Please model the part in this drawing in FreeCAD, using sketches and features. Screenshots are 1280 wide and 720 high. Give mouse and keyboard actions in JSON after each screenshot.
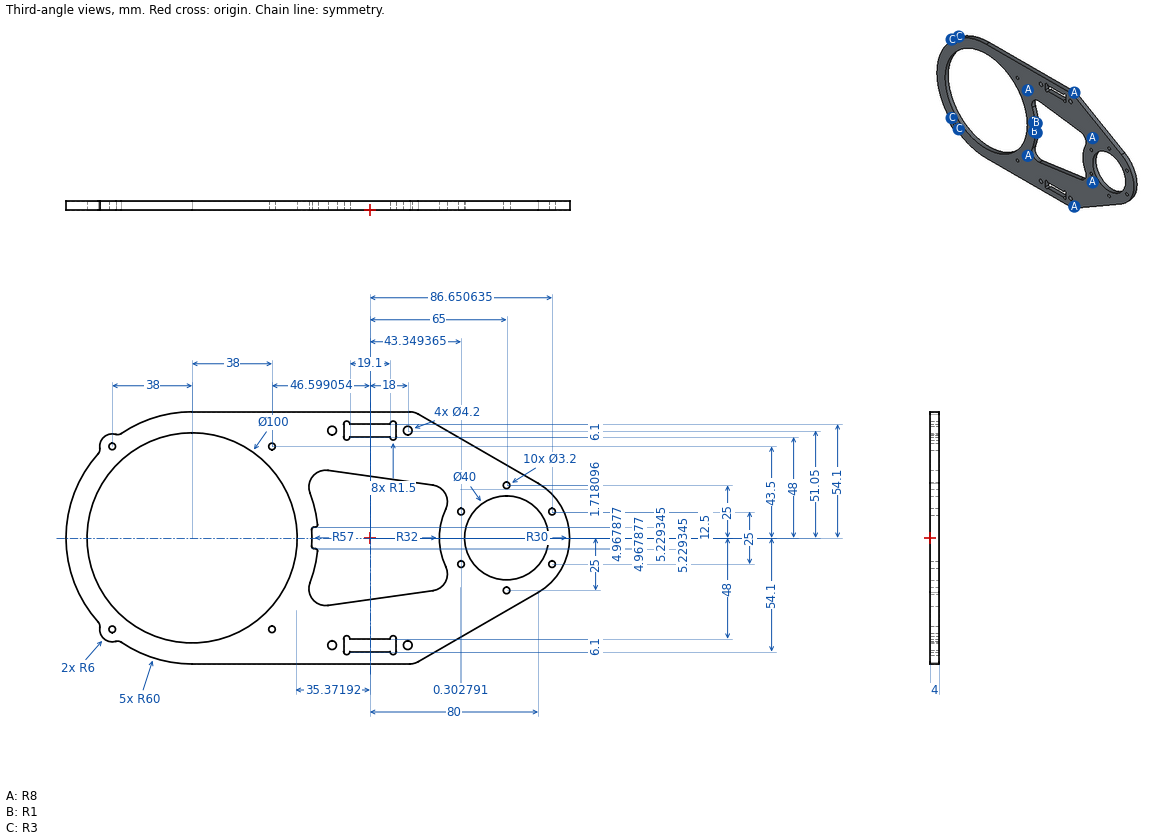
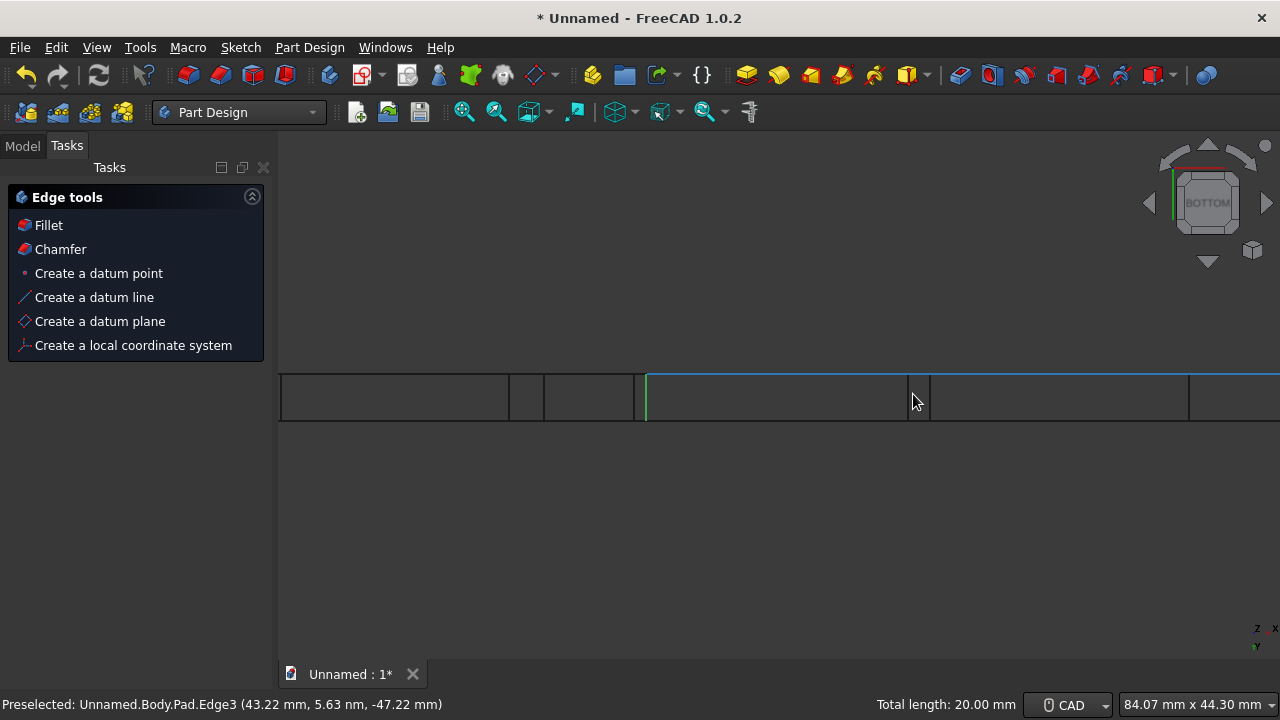
{"action": "left_click", "coordinate": [908, 397], "text": "ctrl"}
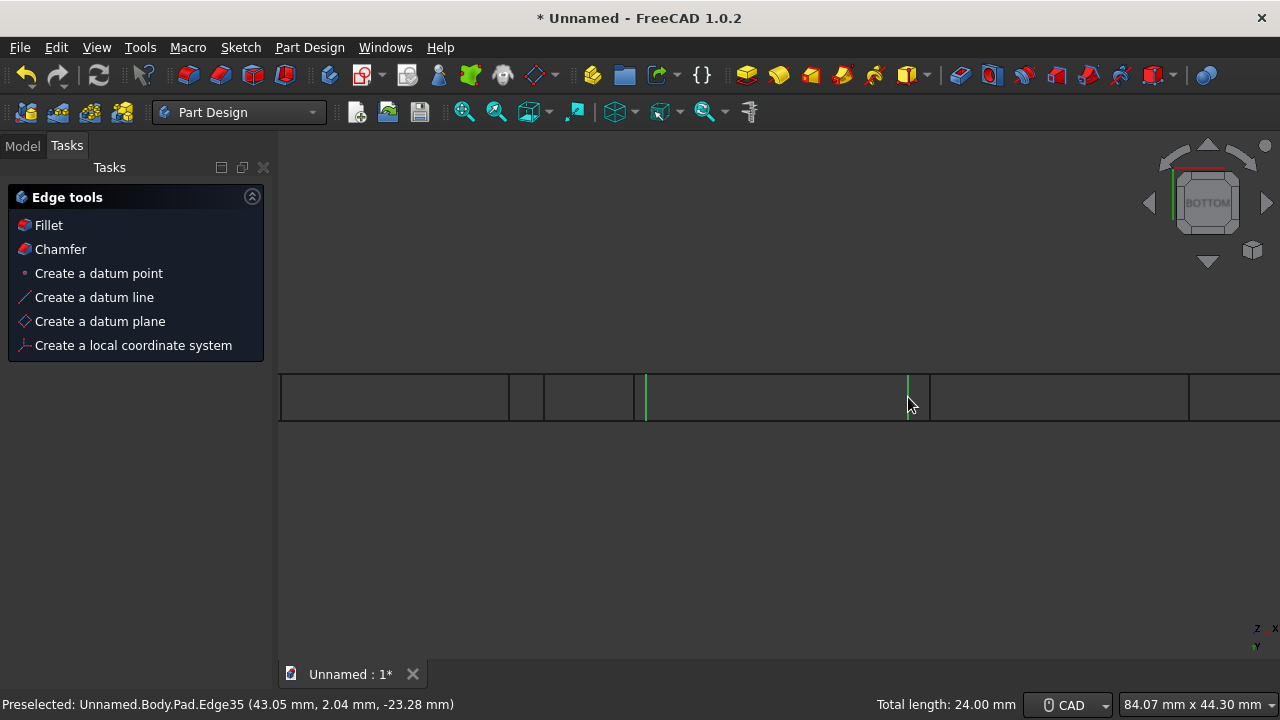
{"action": "key", "text": "v 1"}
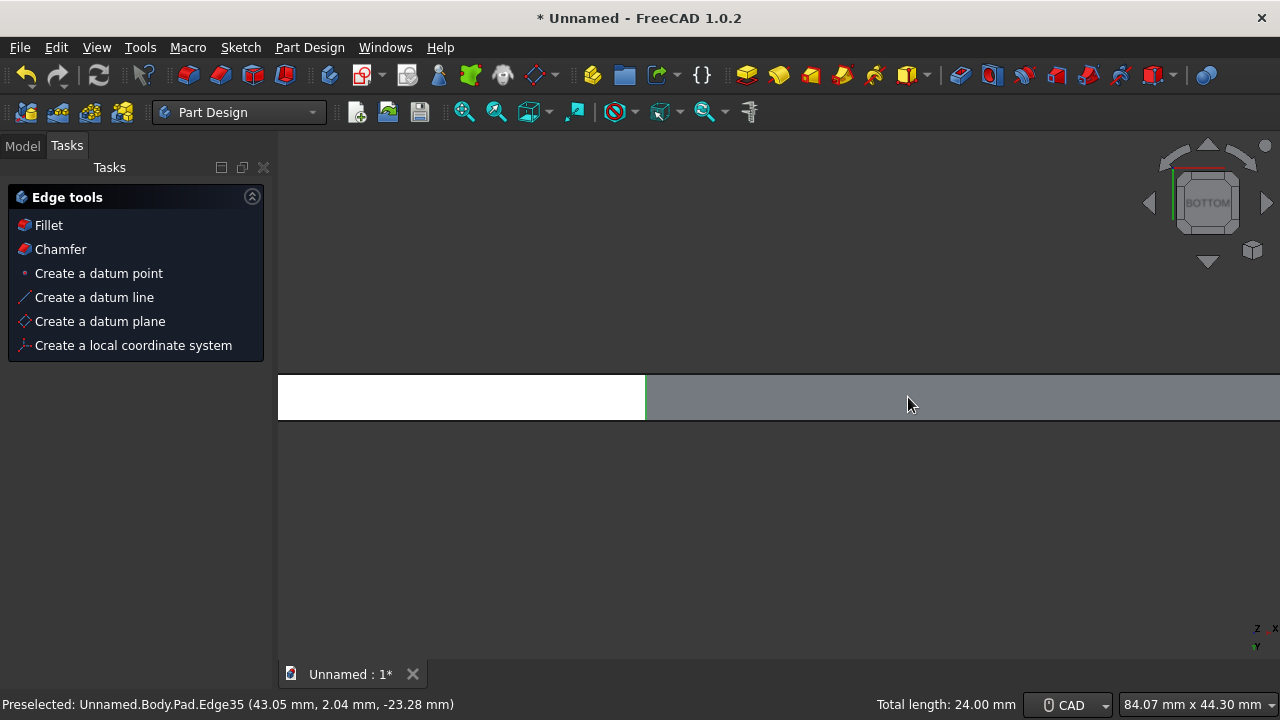
{"action": "left_click", "coordinate": [190, 76]}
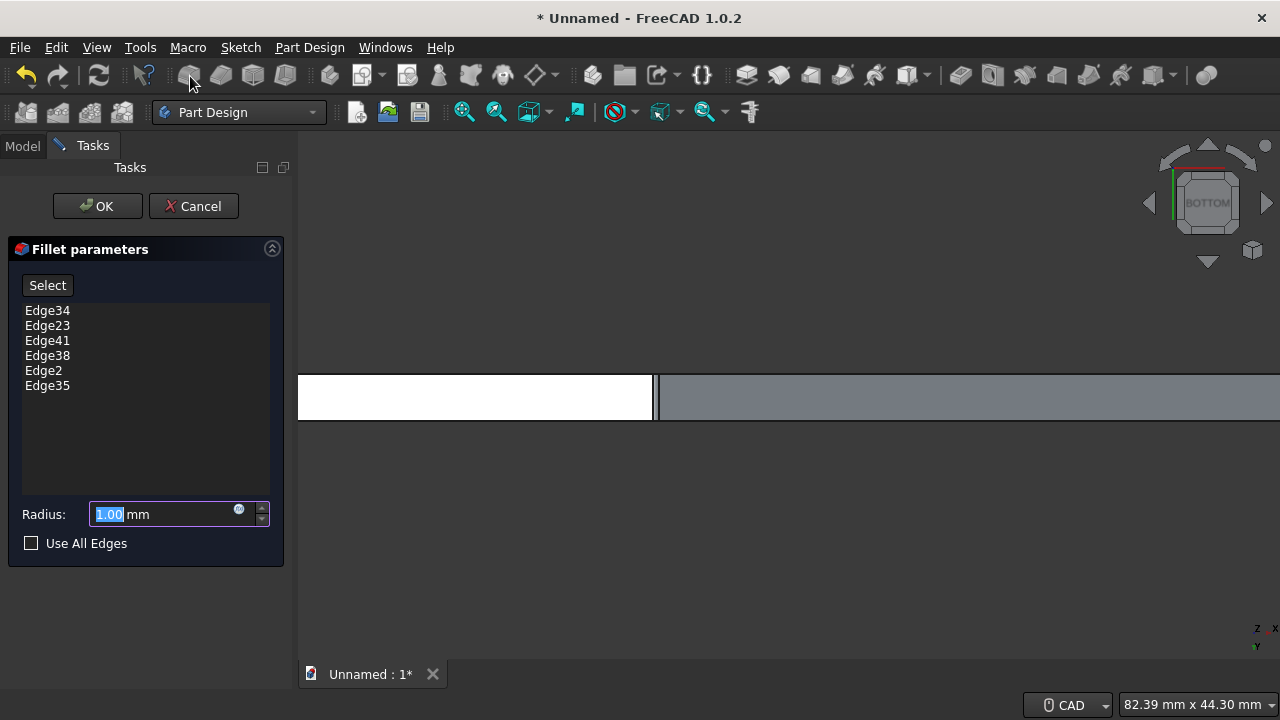
{"action": "type", "text": "8"}
{"action": "key", "text": "Tab"}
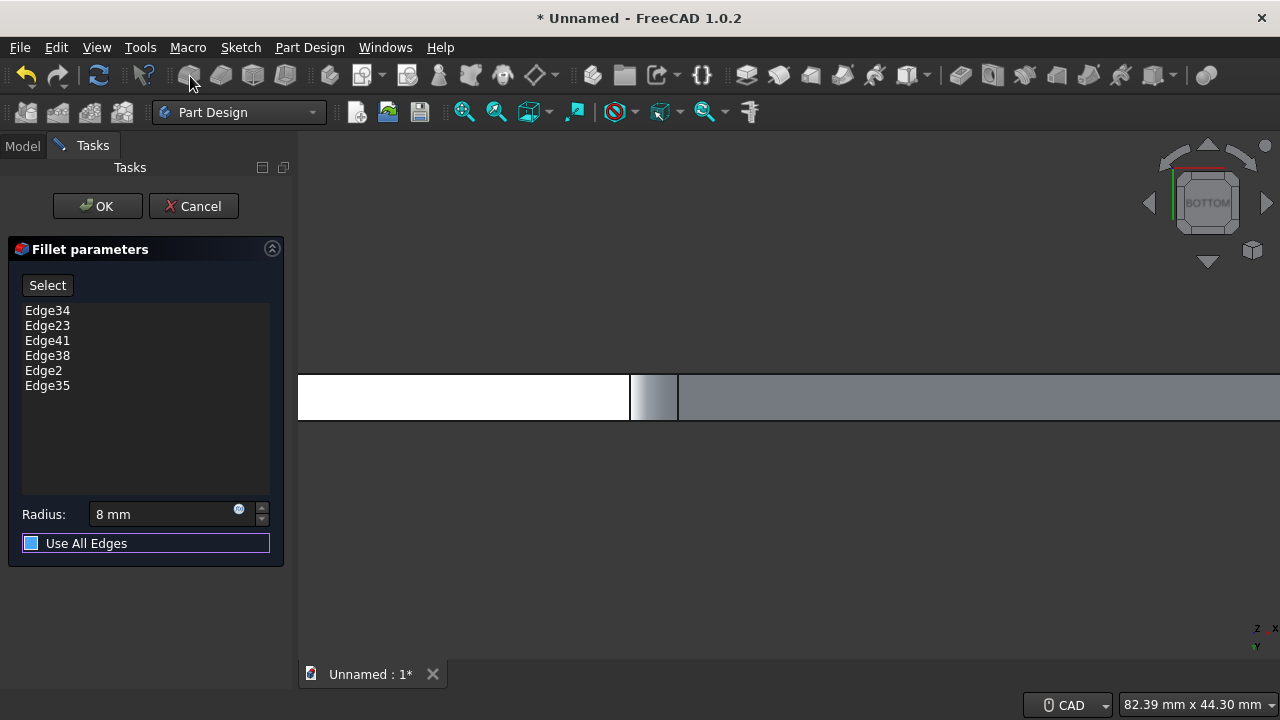
{"action": "left_click", "coordinate": [98, 206]}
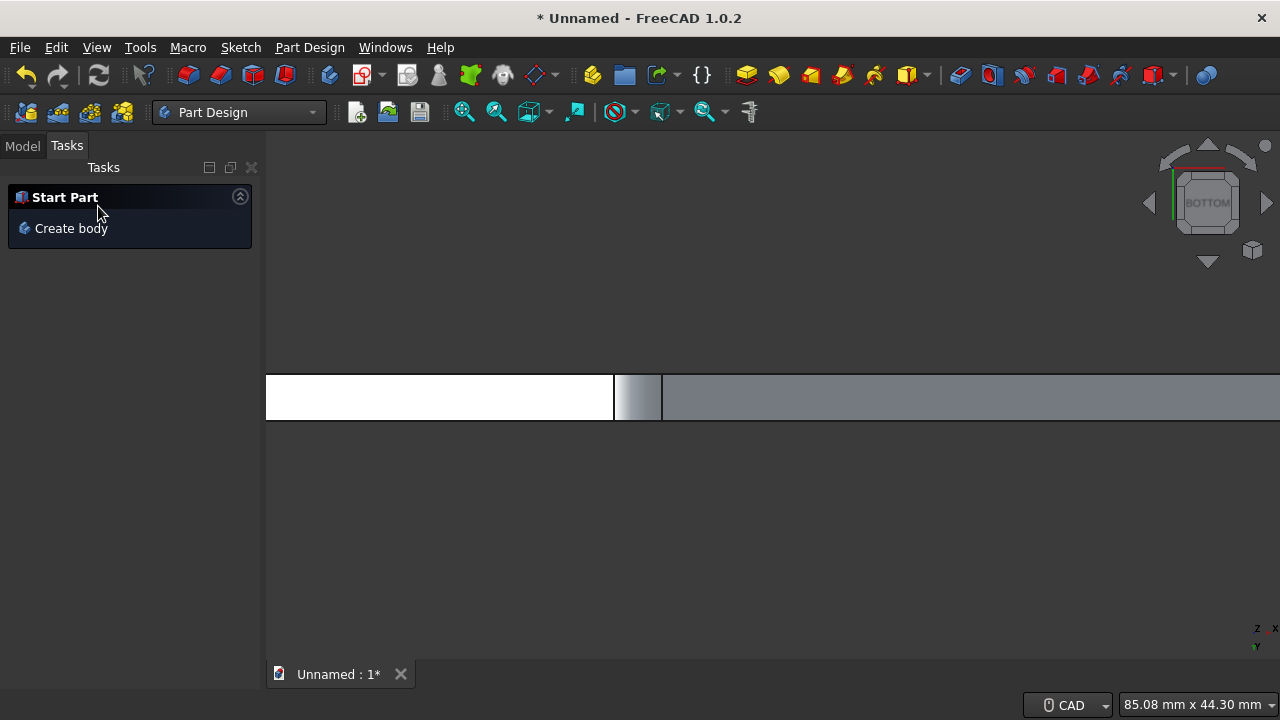
{"action": "left_click", "coordinate": [466, 112]}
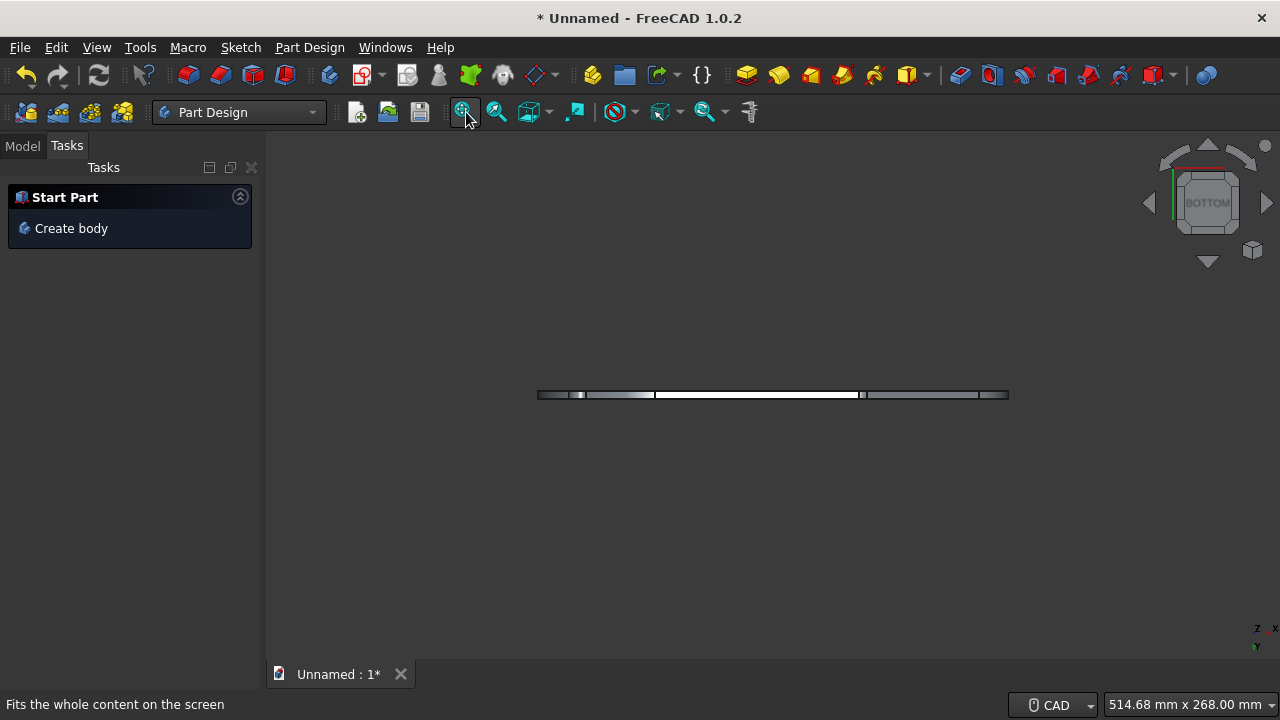
{"action": "scroll", "coordinate": [773, 394], "scroll_direction": "up", "scroll_amount": 9}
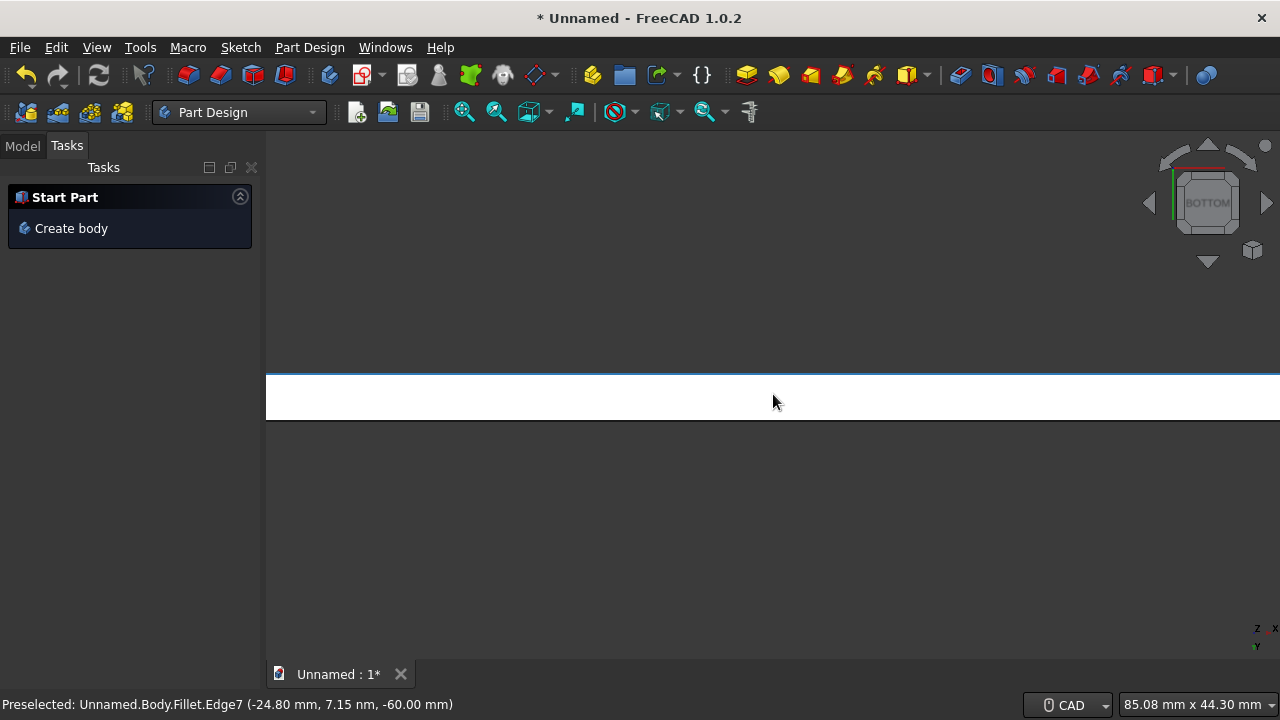
{"action": "left_click", "coordinate": [466, 112]}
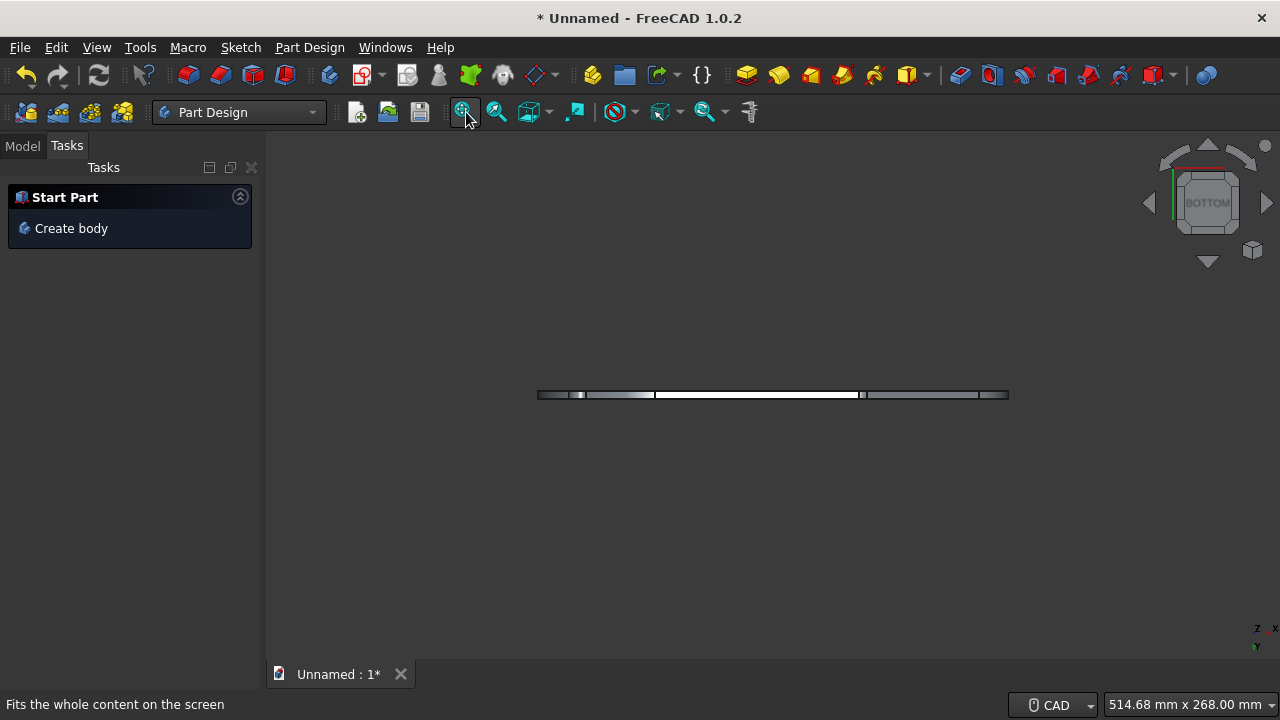
{"action": "key", "text": "0"}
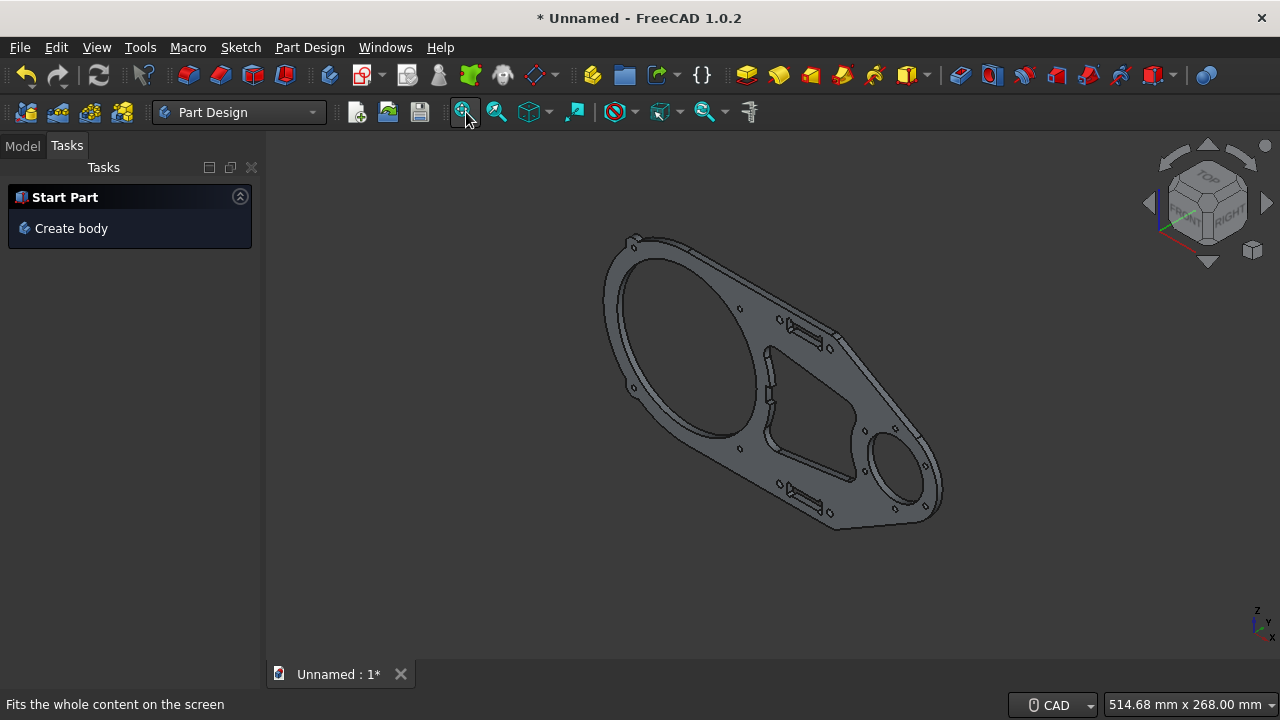
{"action": "scroll", "coordinate": [773, 402], "scroll_direction": "up", "scroll_amount": 9}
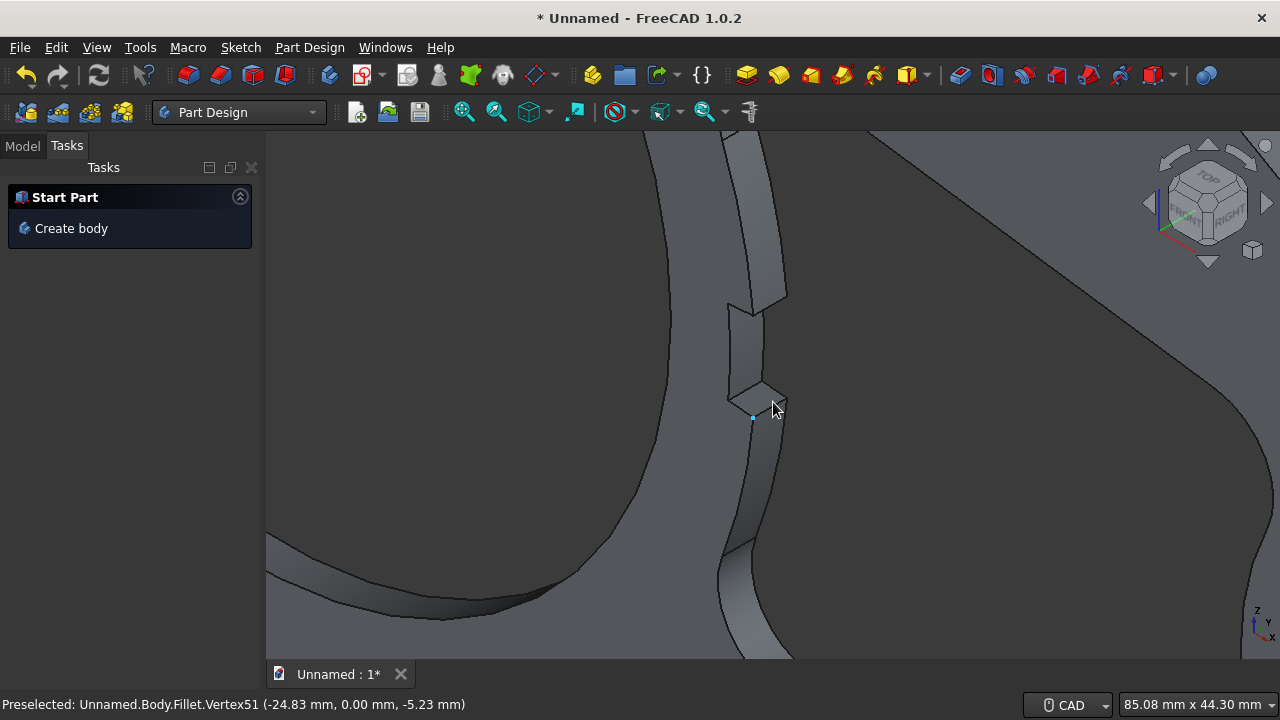
{"action": "left_click", "coordinate": [770, 407]}